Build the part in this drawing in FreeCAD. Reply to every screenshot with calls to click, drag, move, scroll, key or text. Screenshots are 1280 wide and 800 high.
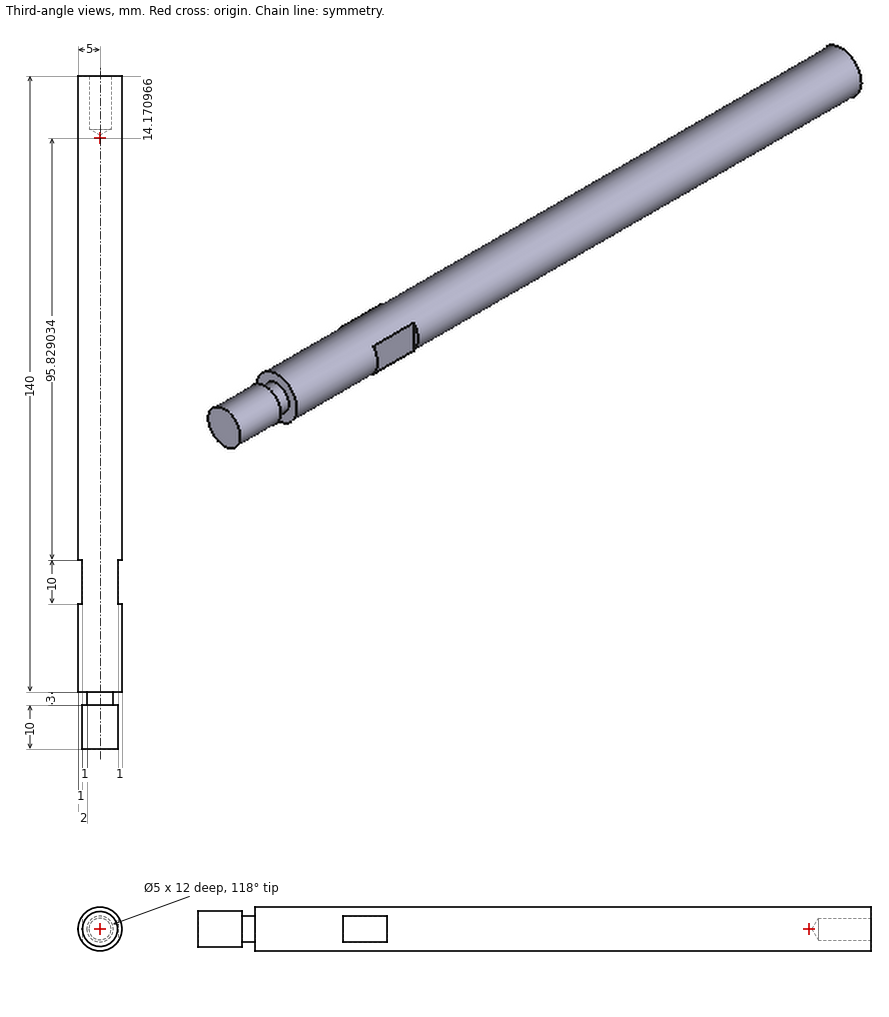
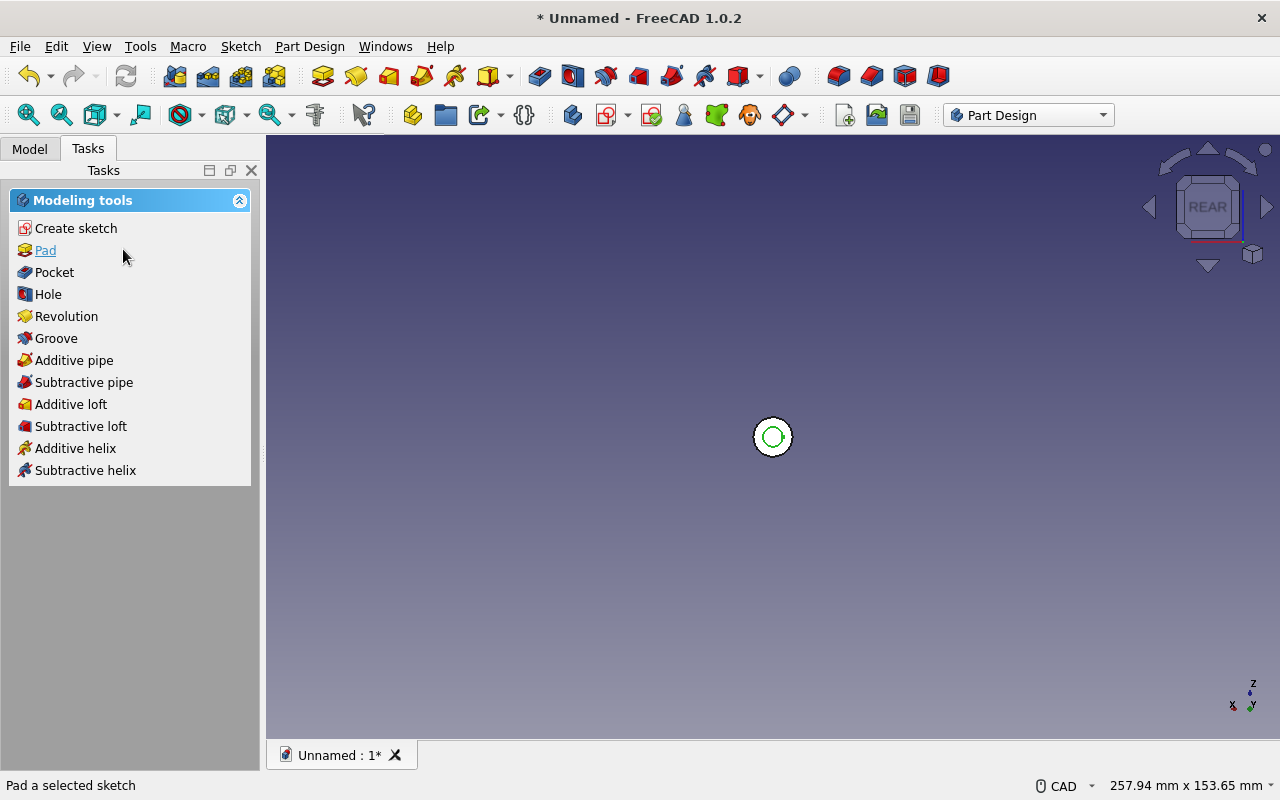
click(573, 76)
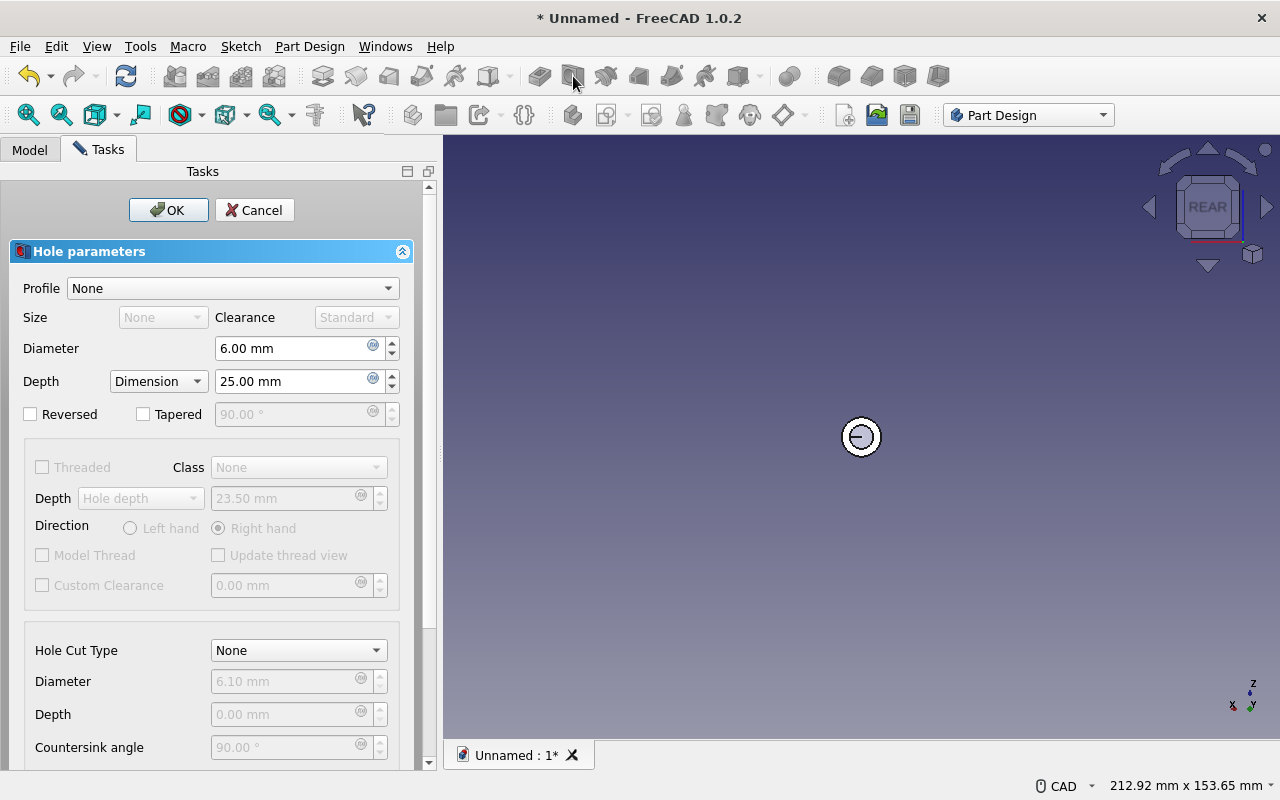
triple_click(300, 348)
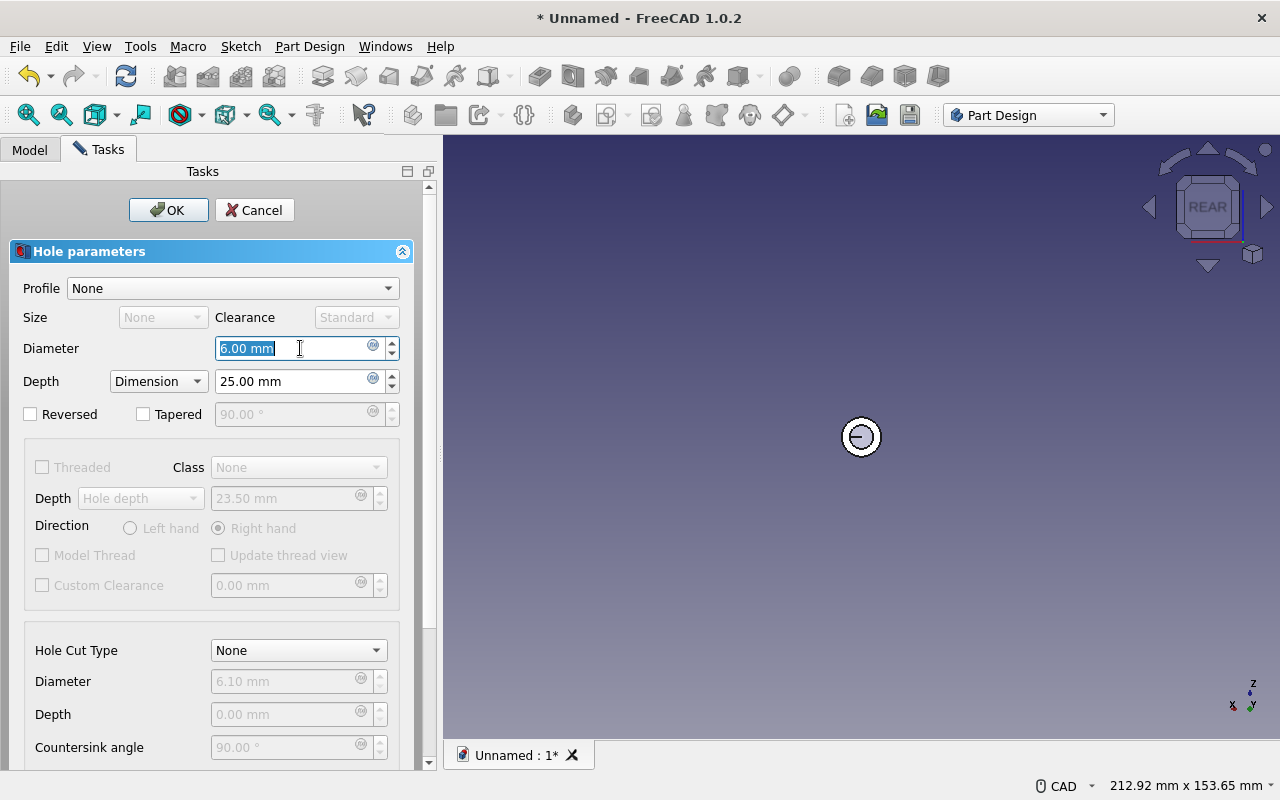
text(5)
key(Tab)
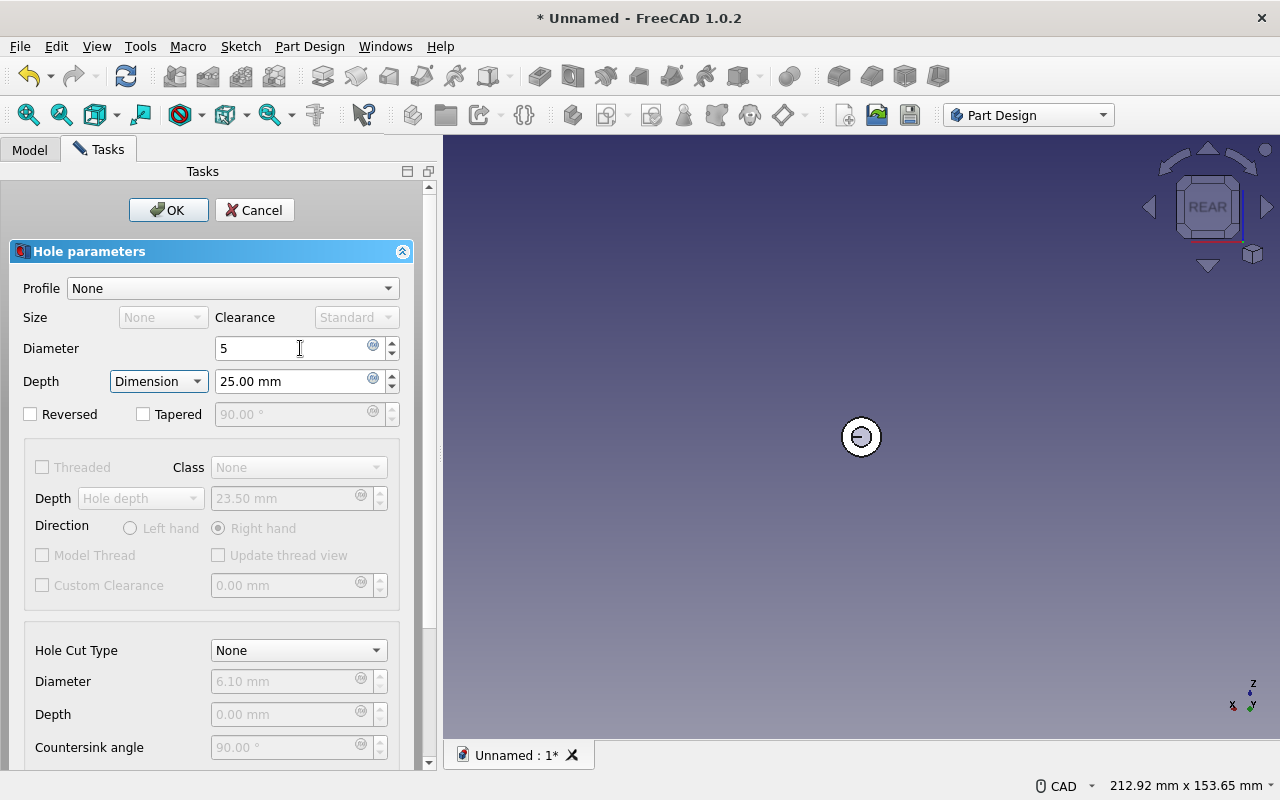
triple_click(300, 382)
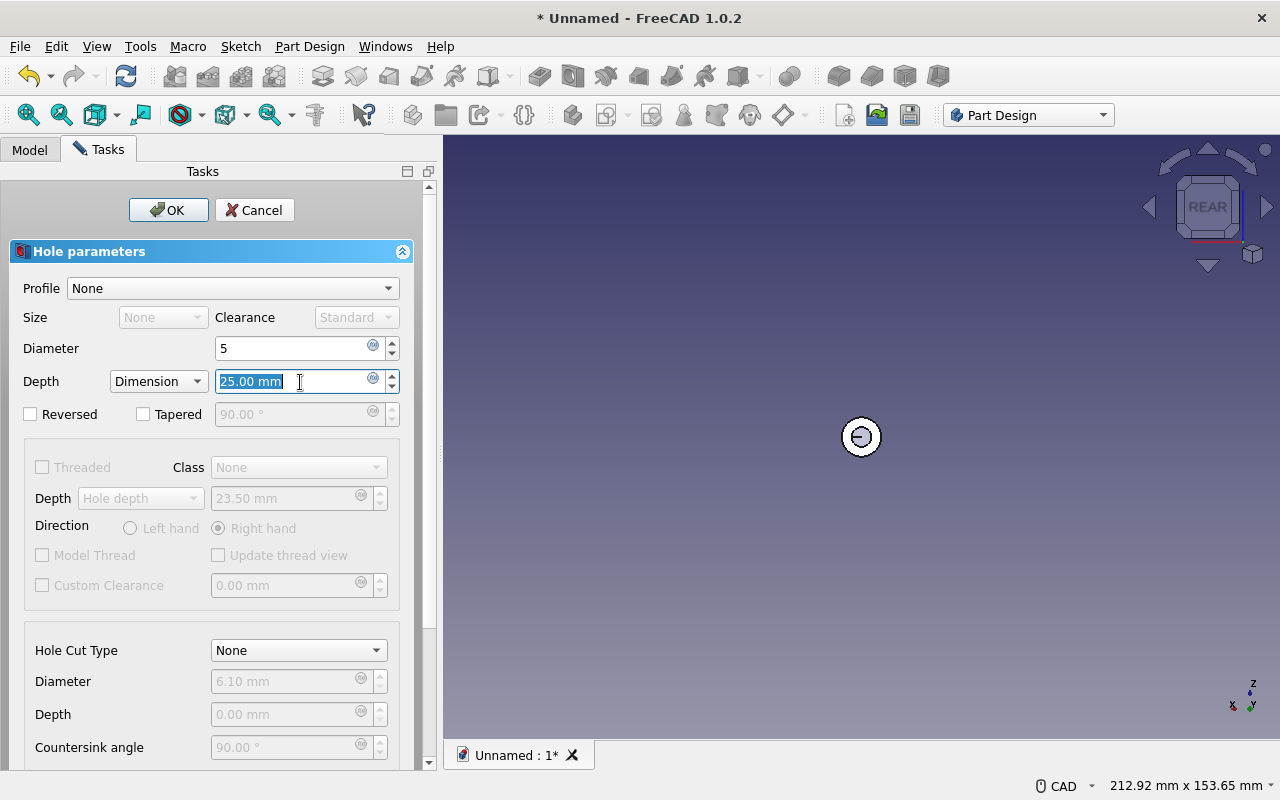
text(12)
key(Tab)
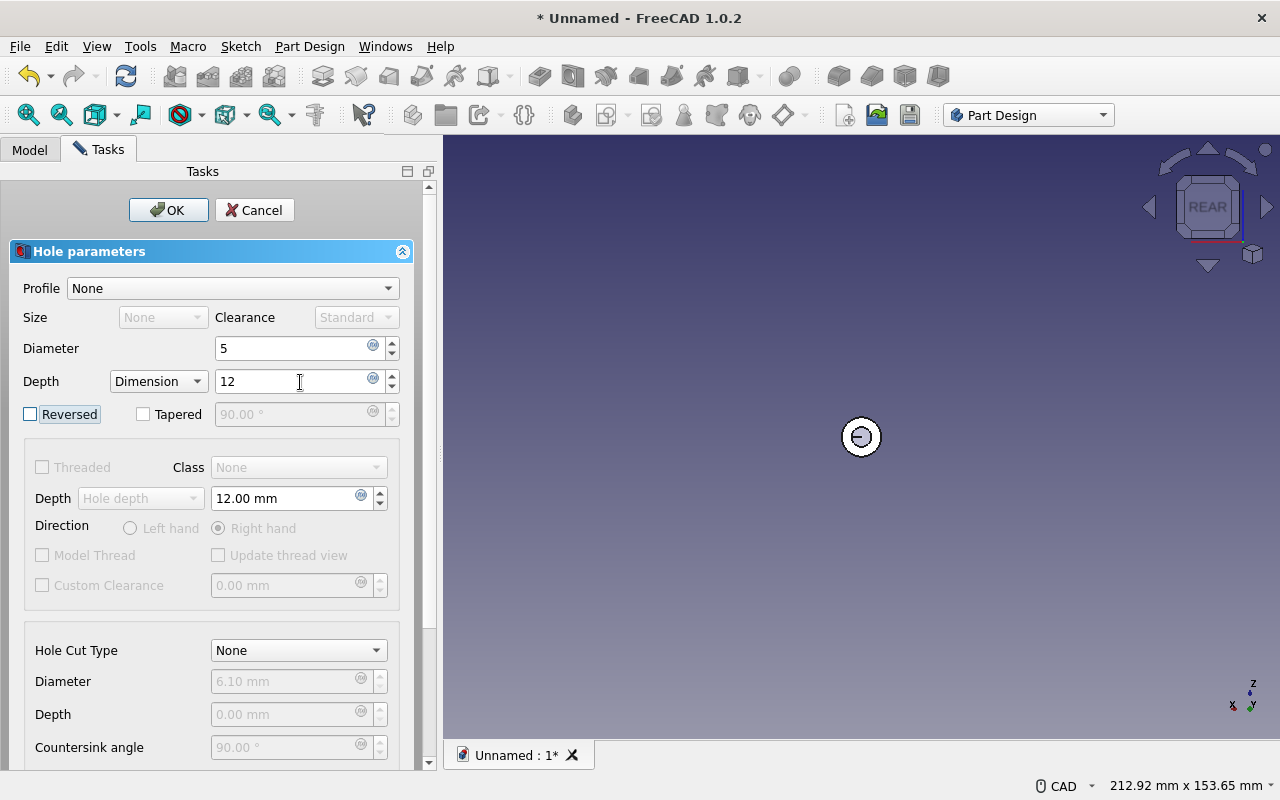
click(169, 210)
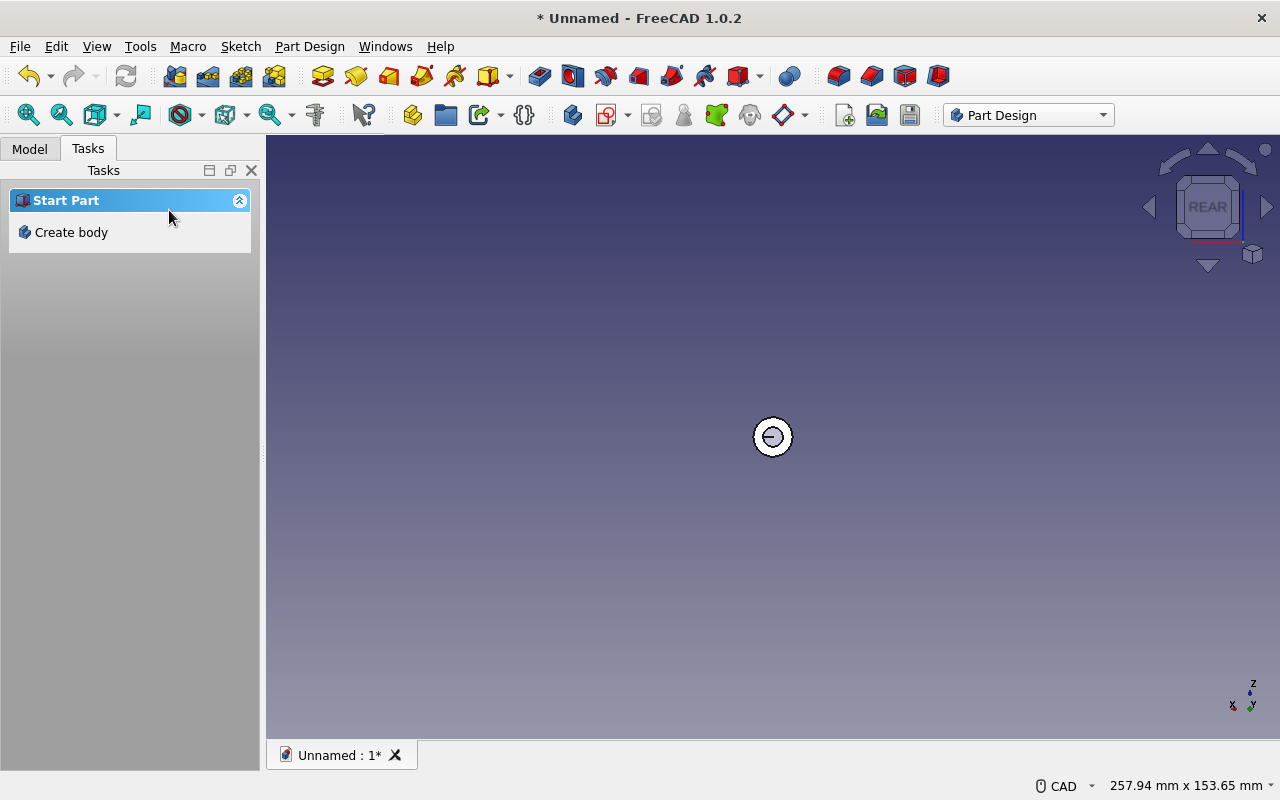
key(0)